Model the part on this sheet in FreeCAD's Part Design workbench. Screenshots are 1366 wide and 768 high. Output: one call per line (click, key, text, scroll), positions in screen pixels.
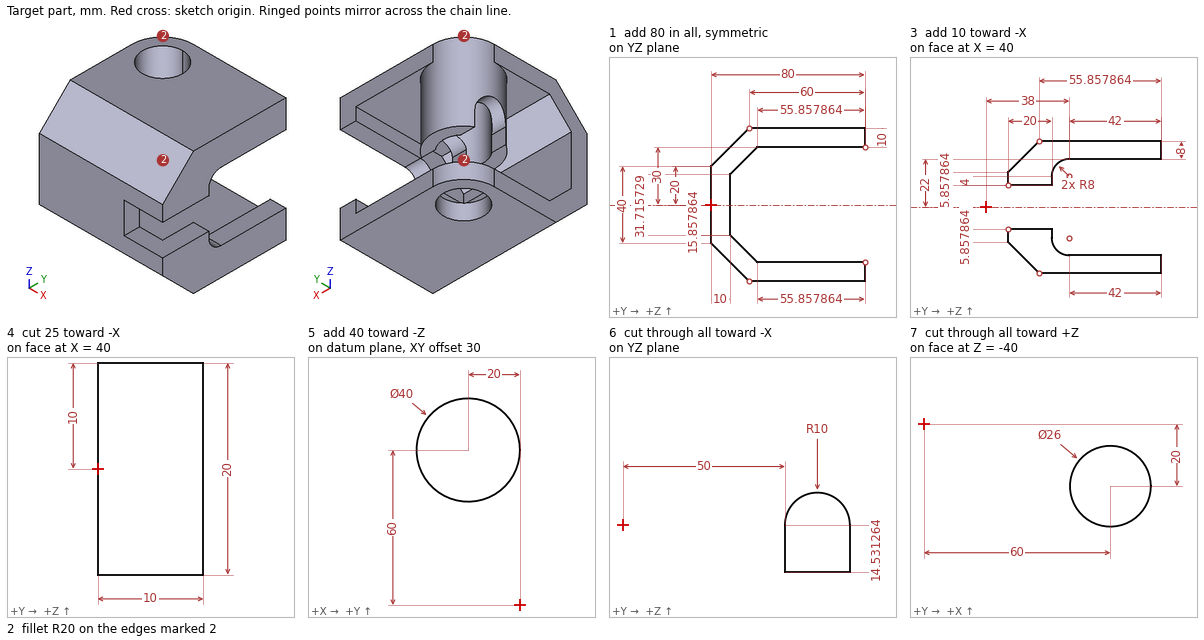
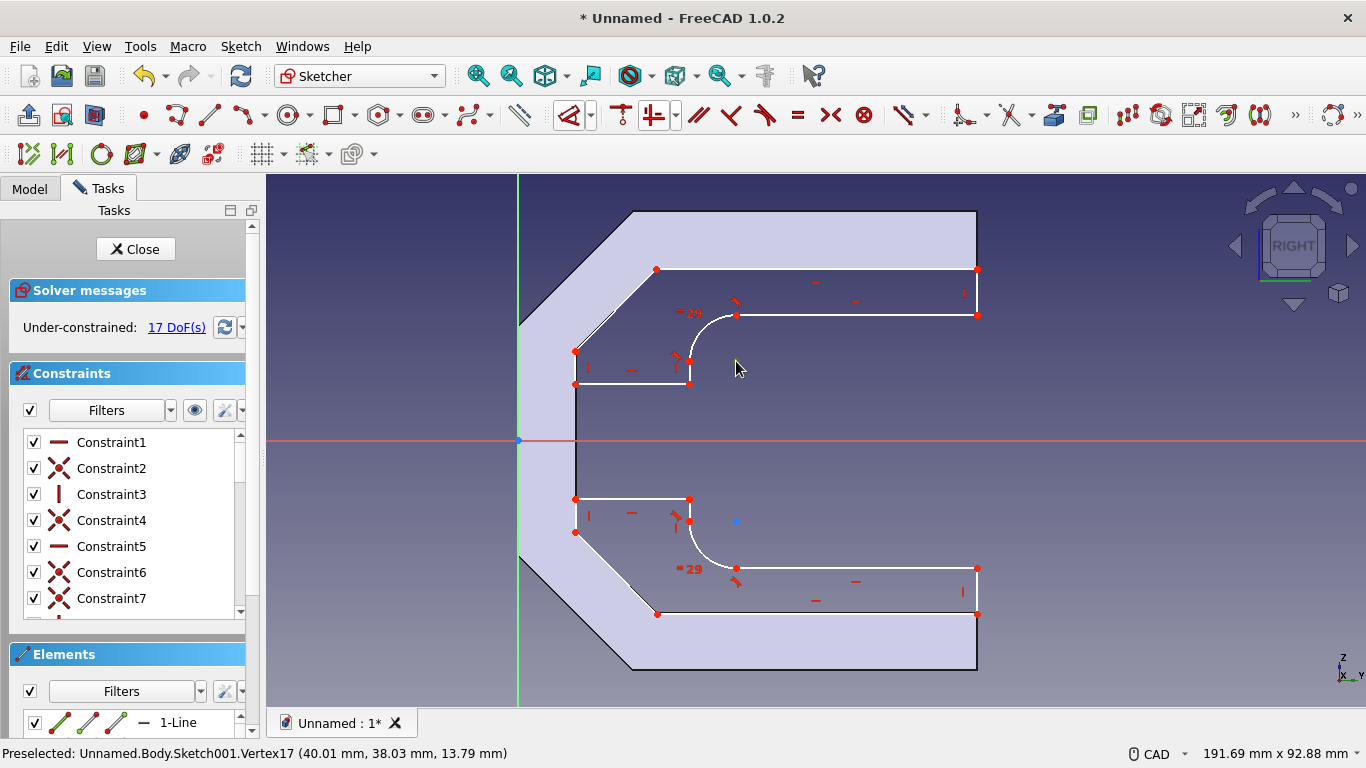
click(736, 522)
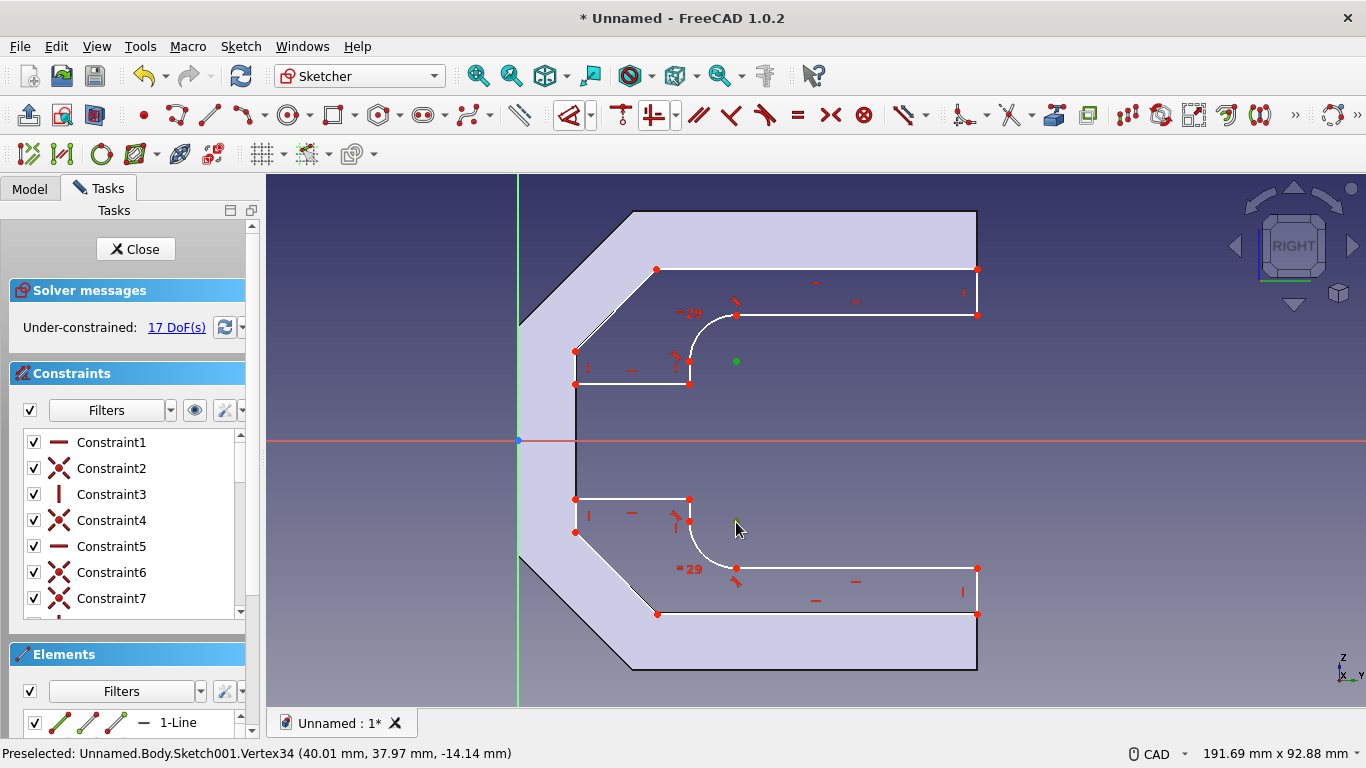
click(359, 441)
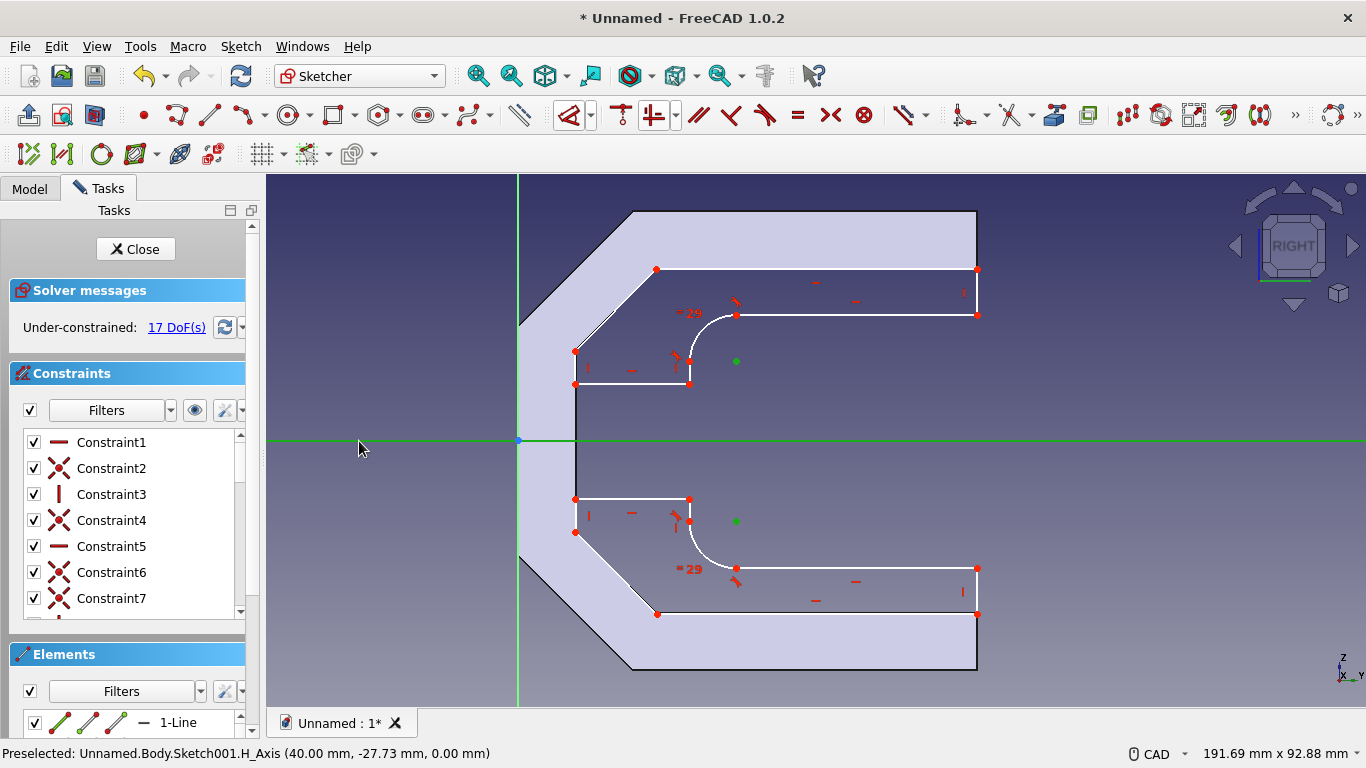
click(831, 116)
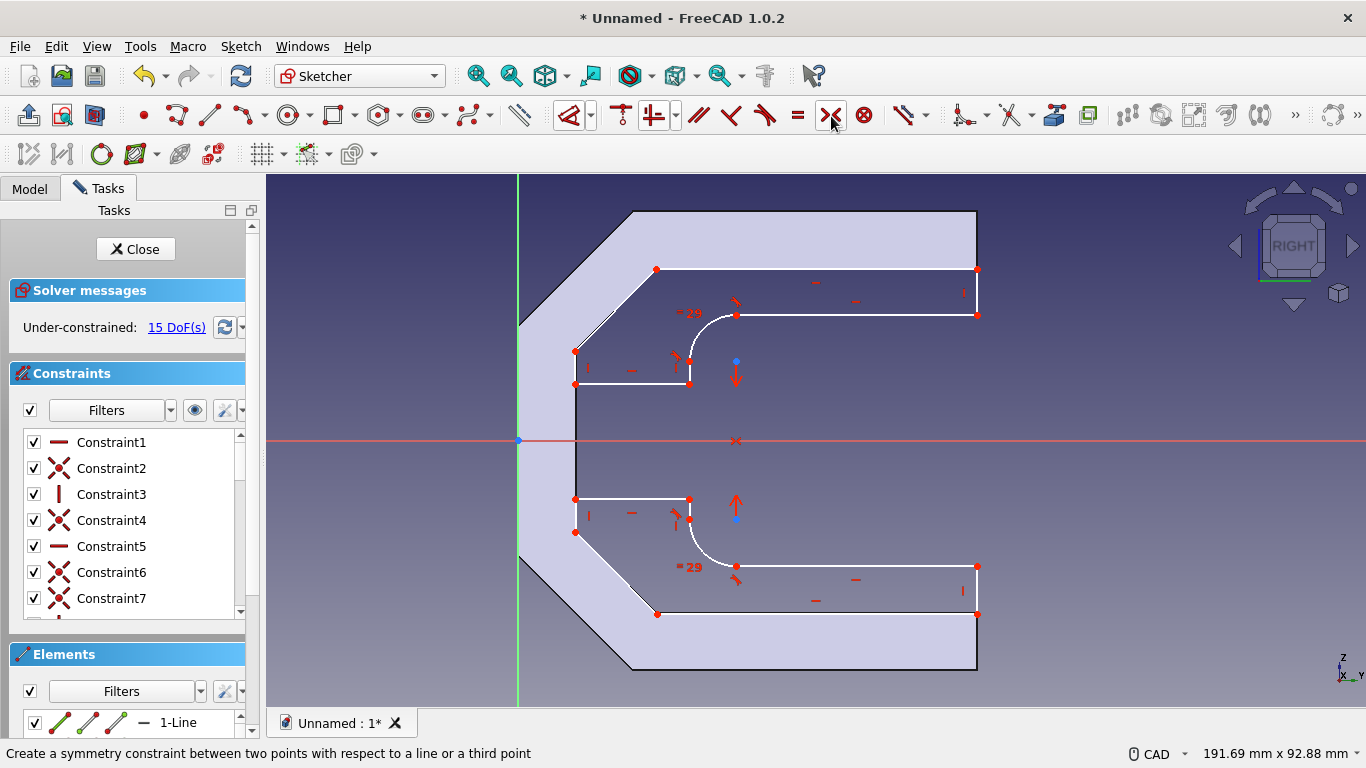
click(575, 384)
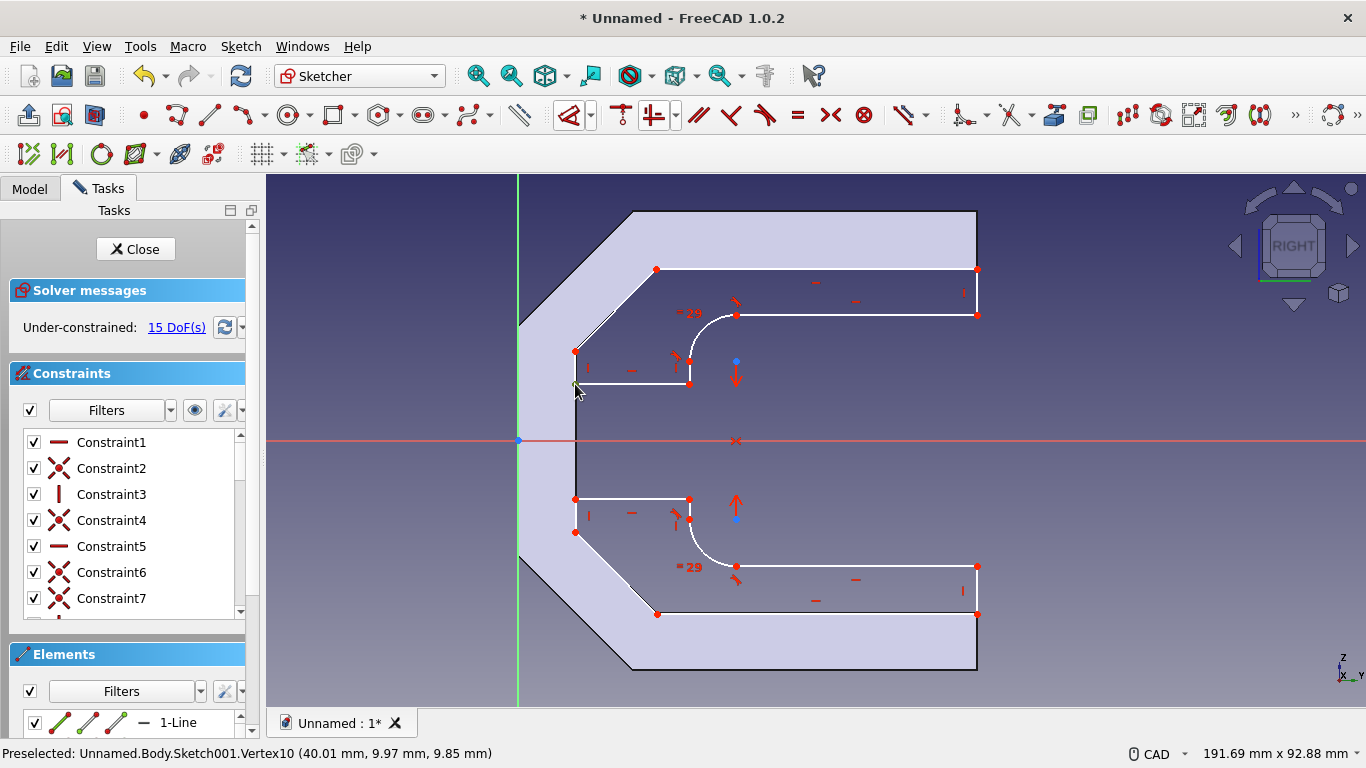
click(576, 499)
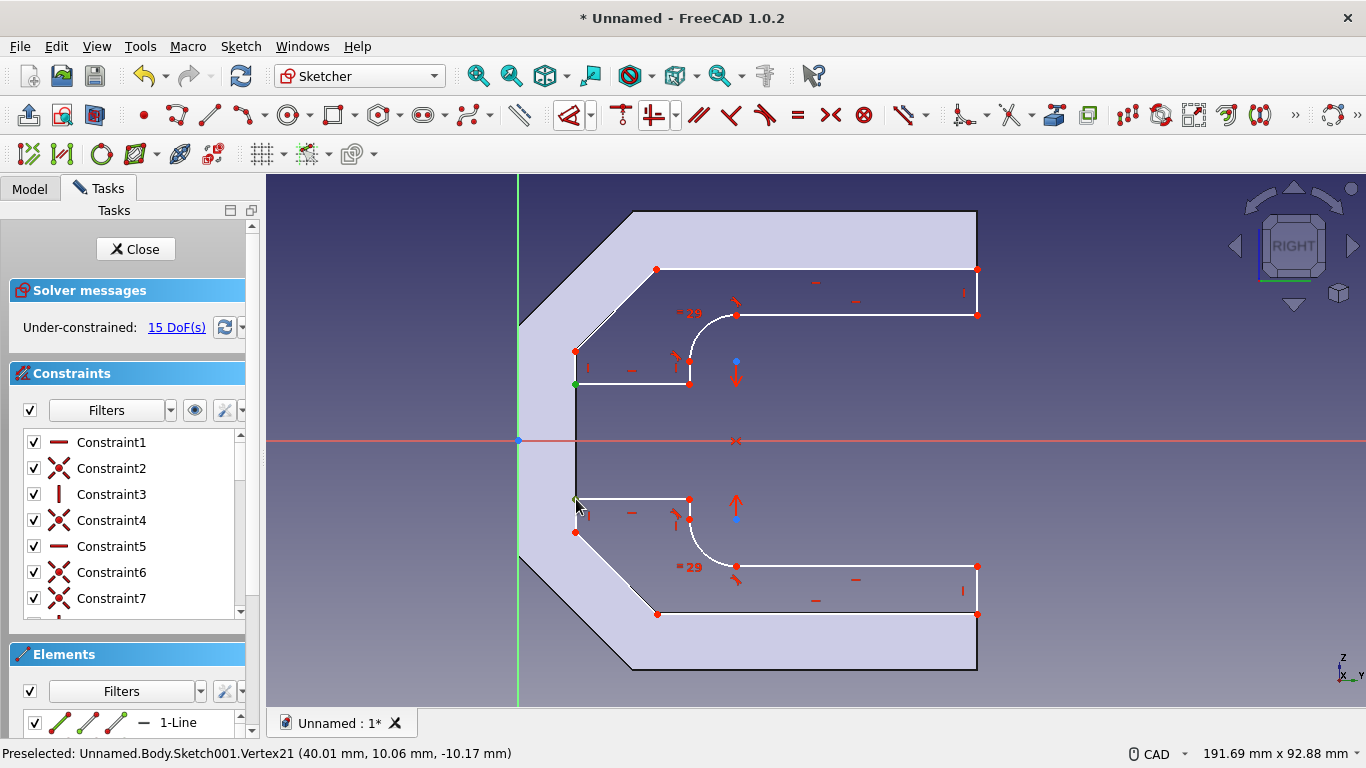
click(359, 441)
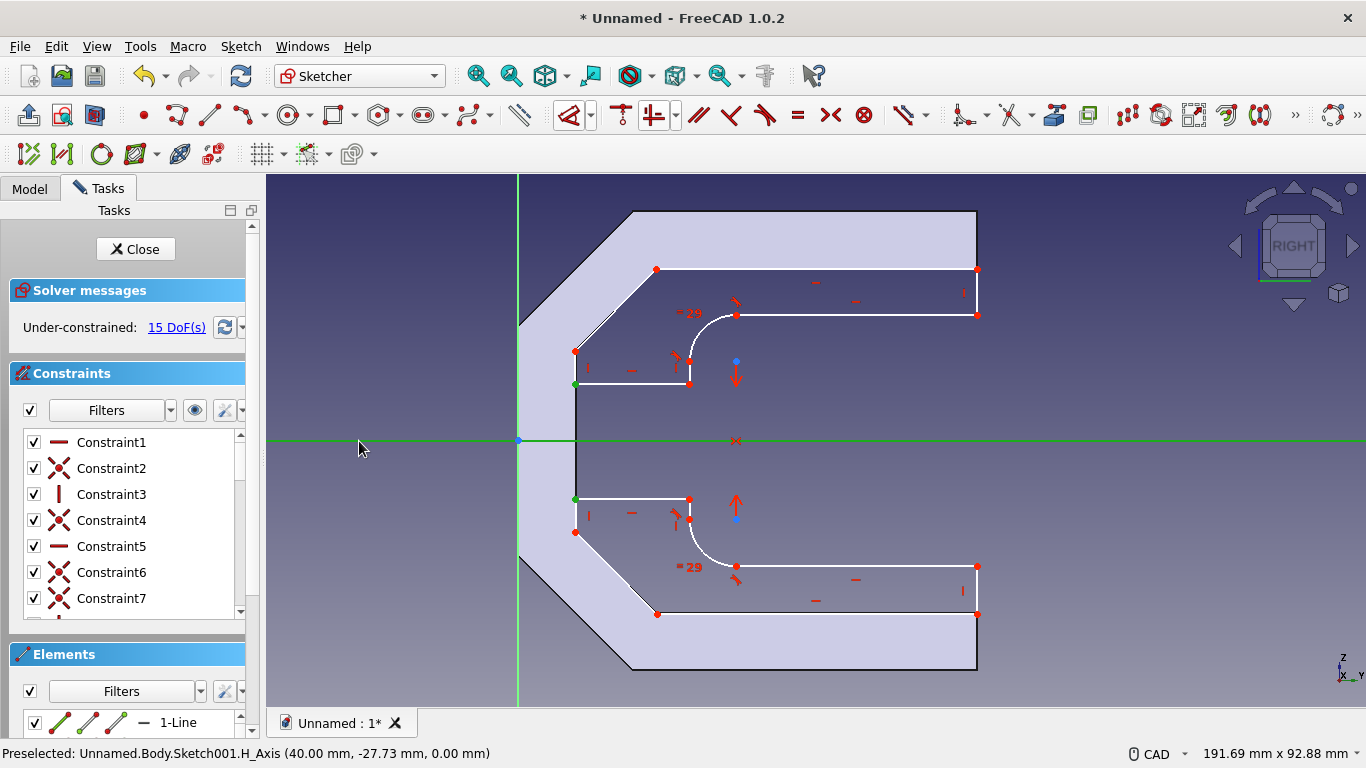
click(831, 116)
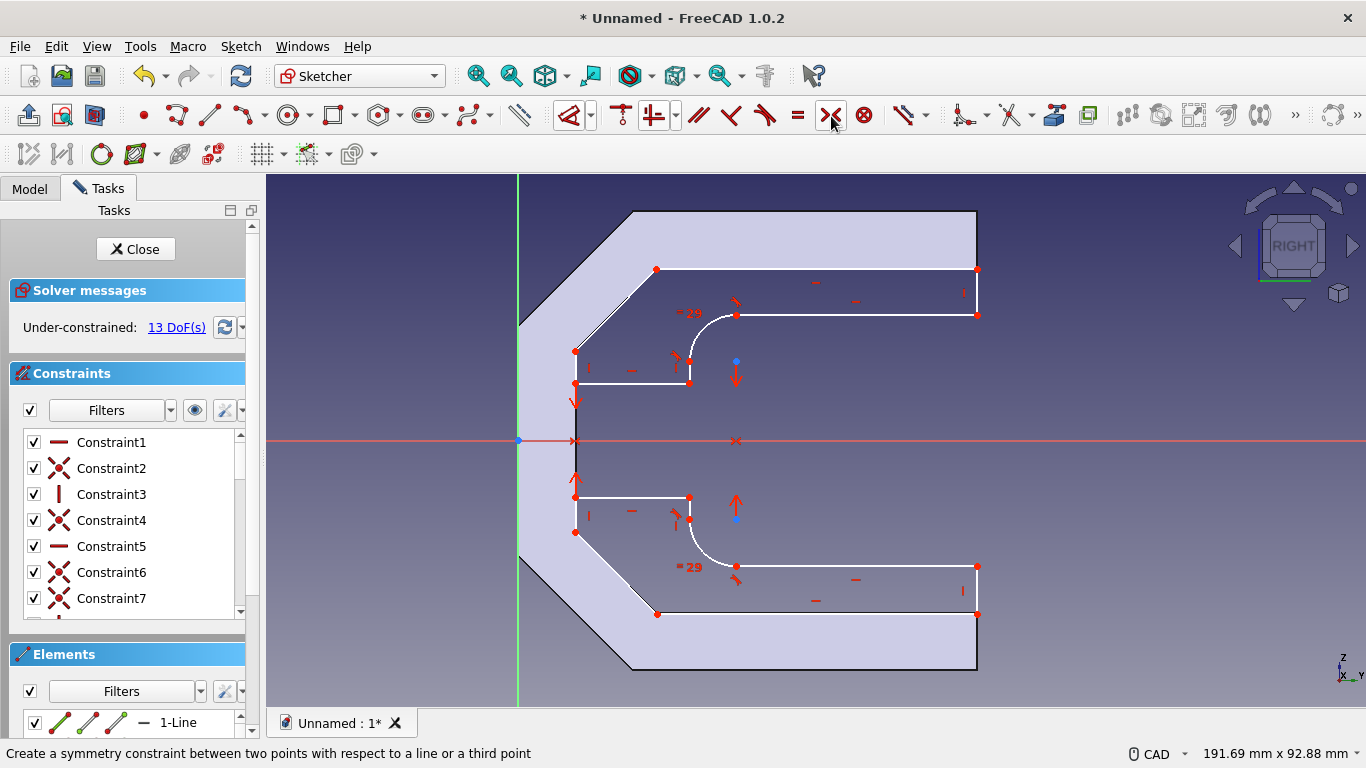
click(656, 269)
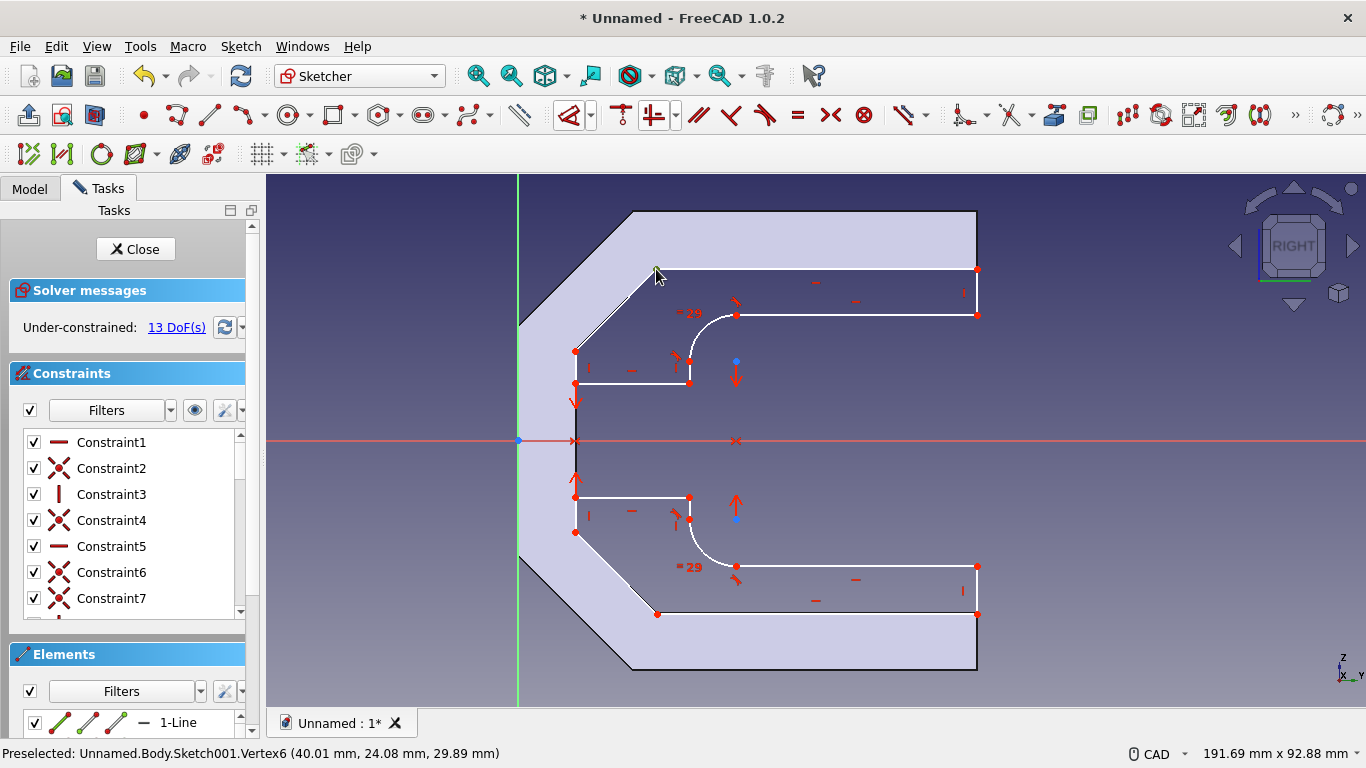
click(657, 614)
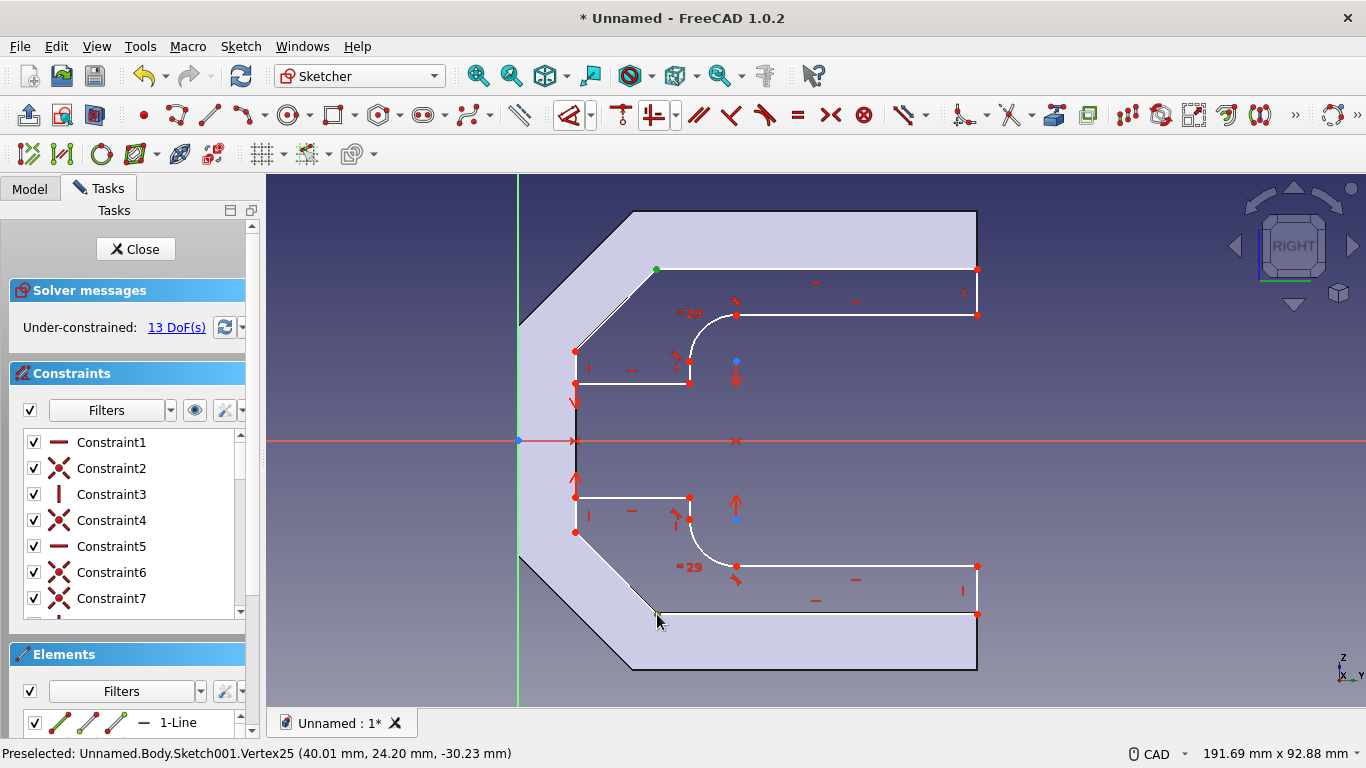
click(359, 441)